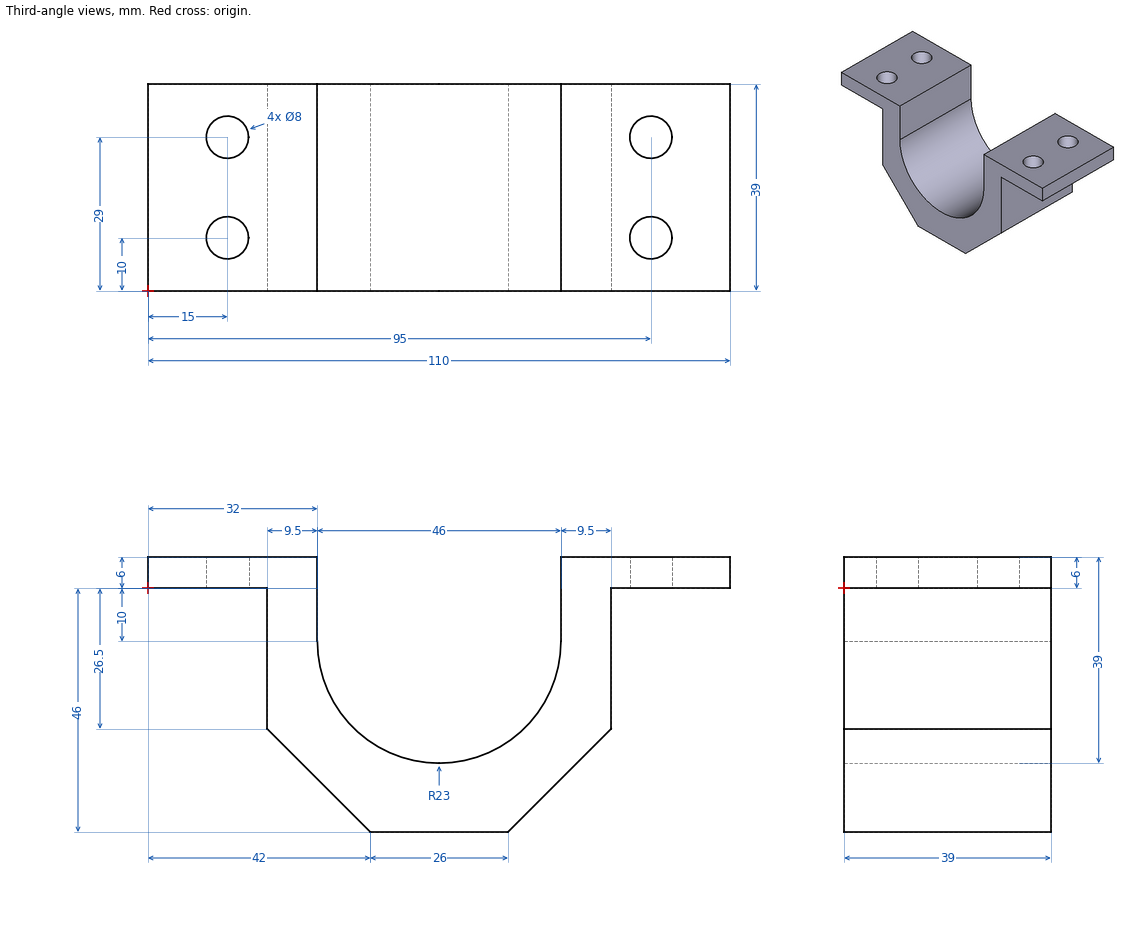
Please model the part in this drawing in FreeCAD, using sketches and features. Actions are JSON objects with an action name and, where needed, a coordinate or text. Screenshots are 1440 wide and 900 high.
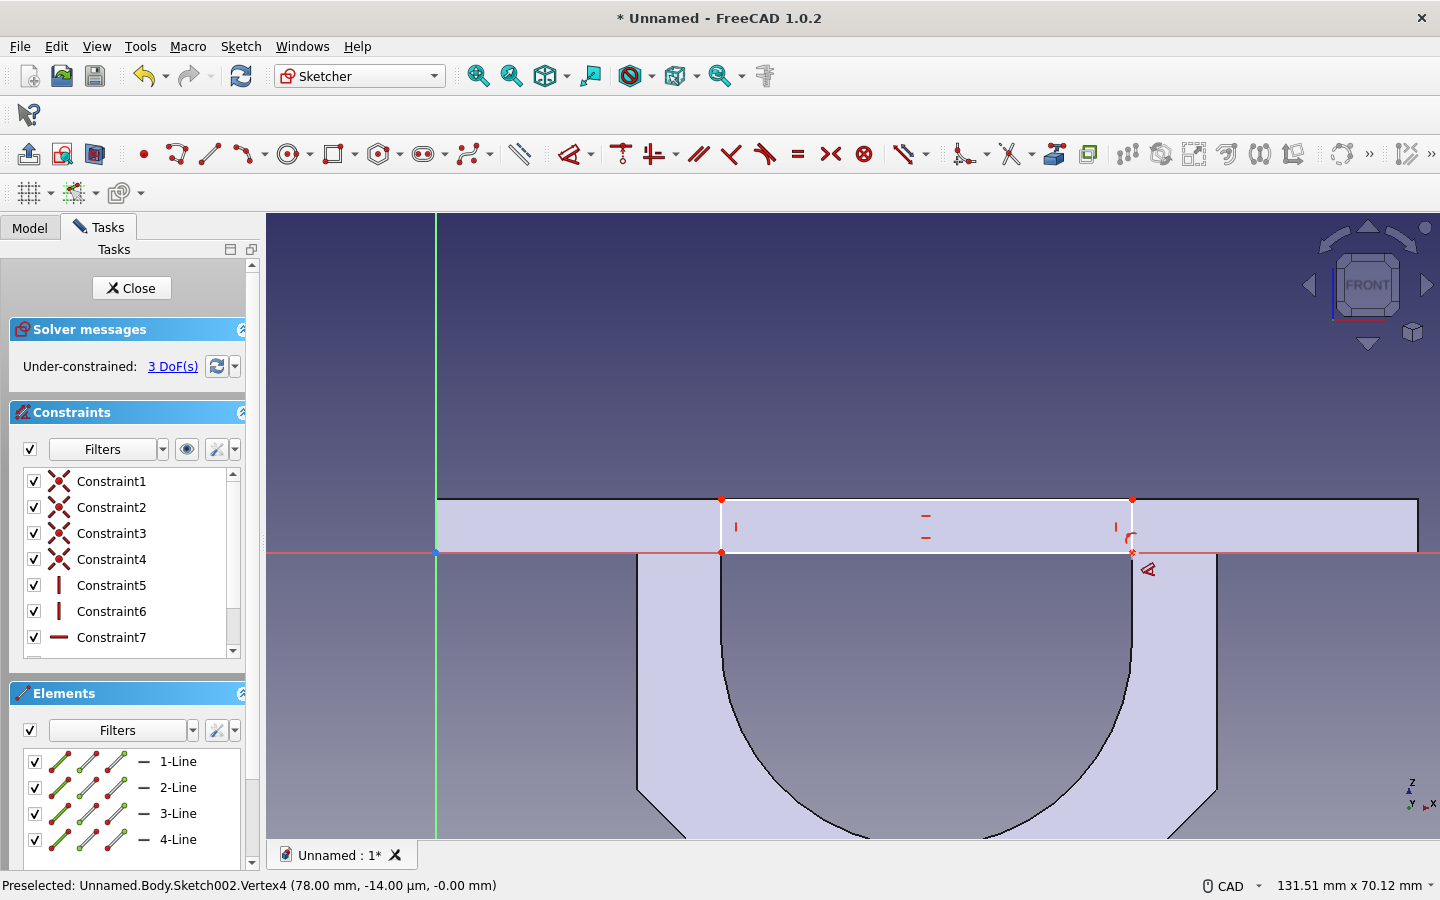
{"action": "left_click", "coordinate": [721, 516]}
{"action": "left_click", "coordinate": [687, 526]}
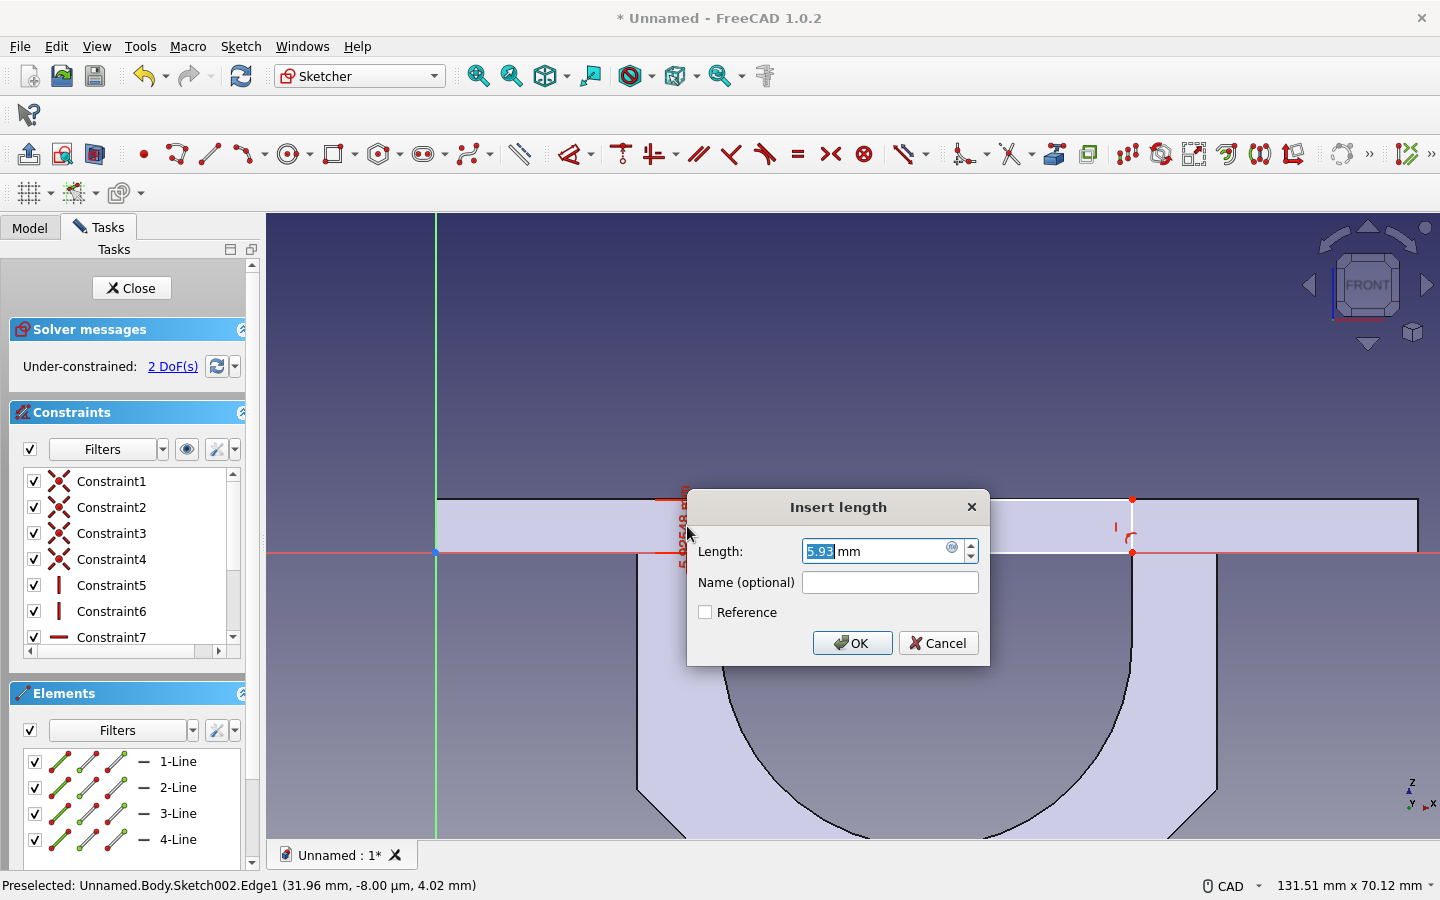
{"action": "type", "text": "6"}
{"action": "key", "text": "Return"}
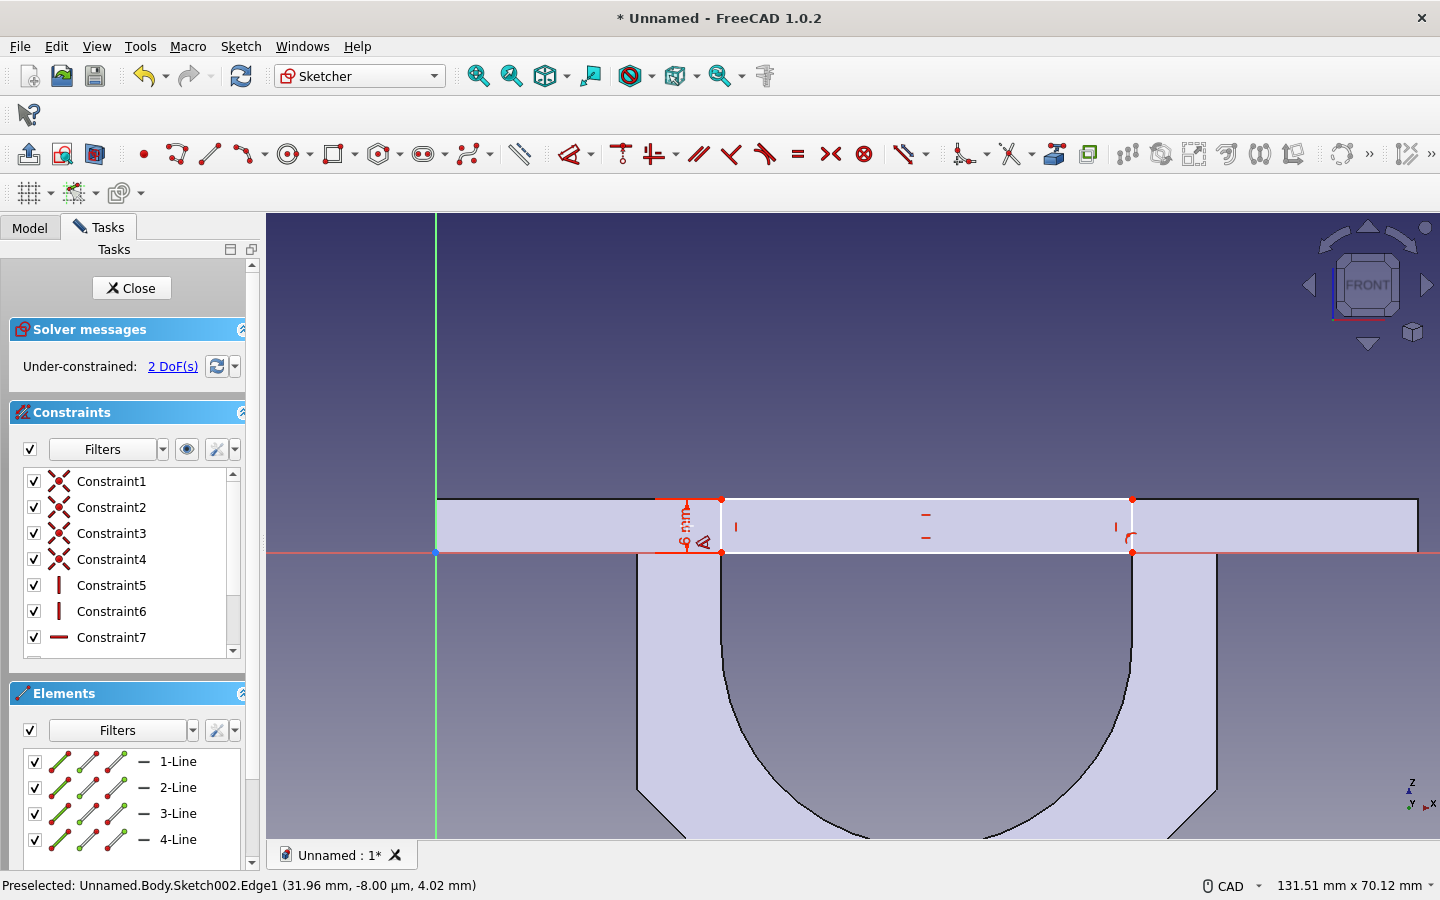
{"action": "left_click", "coordinate": [844, 553]}
{"action": "left_click", "coordinate": [926, 587]}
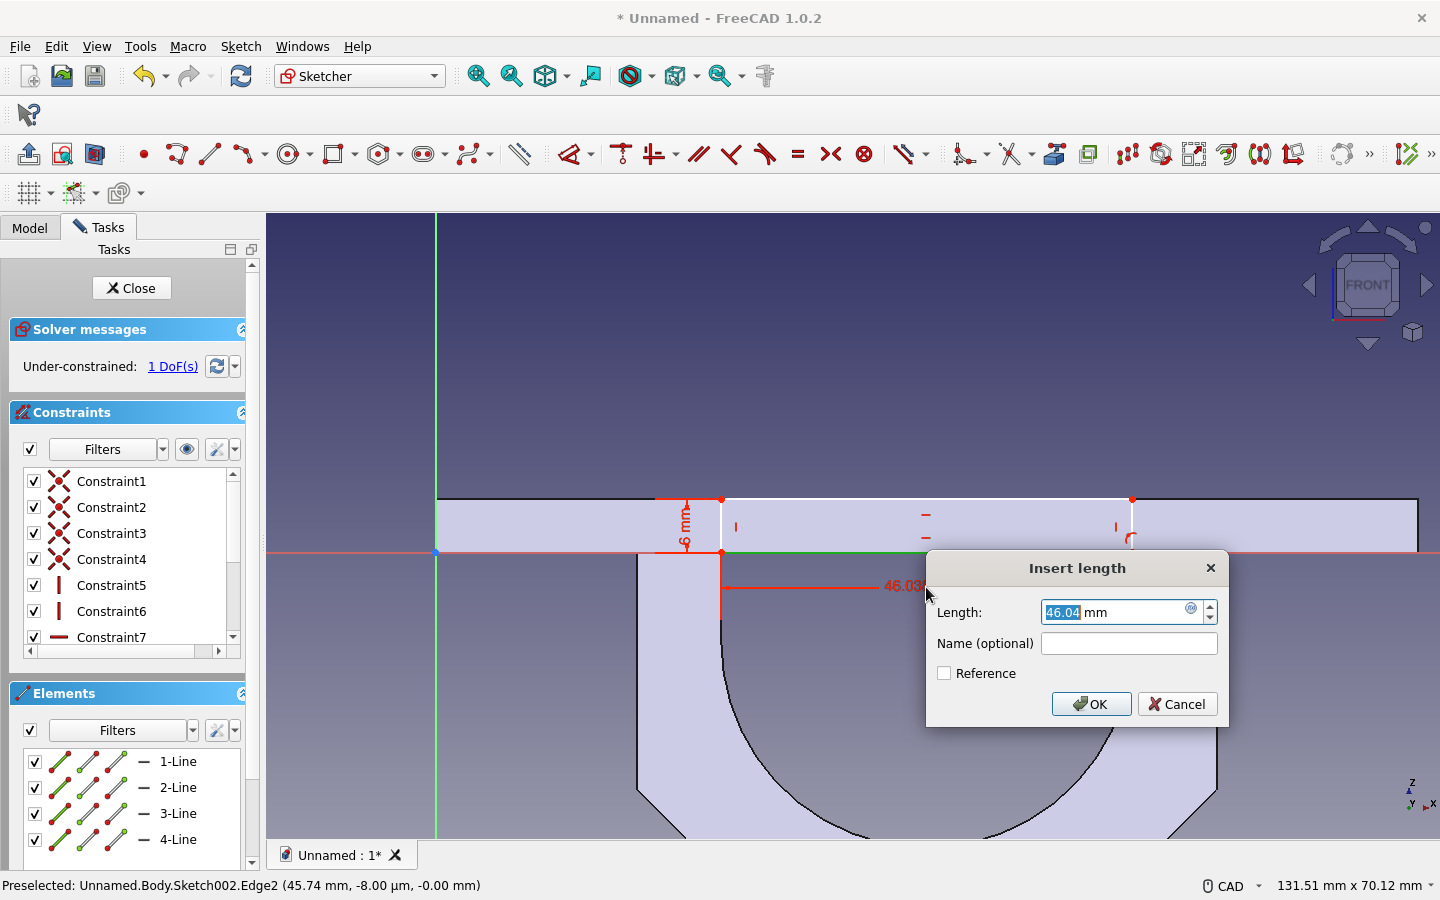
{"action": "type", "text": "46"}
{"action": "key", "text": "Return"}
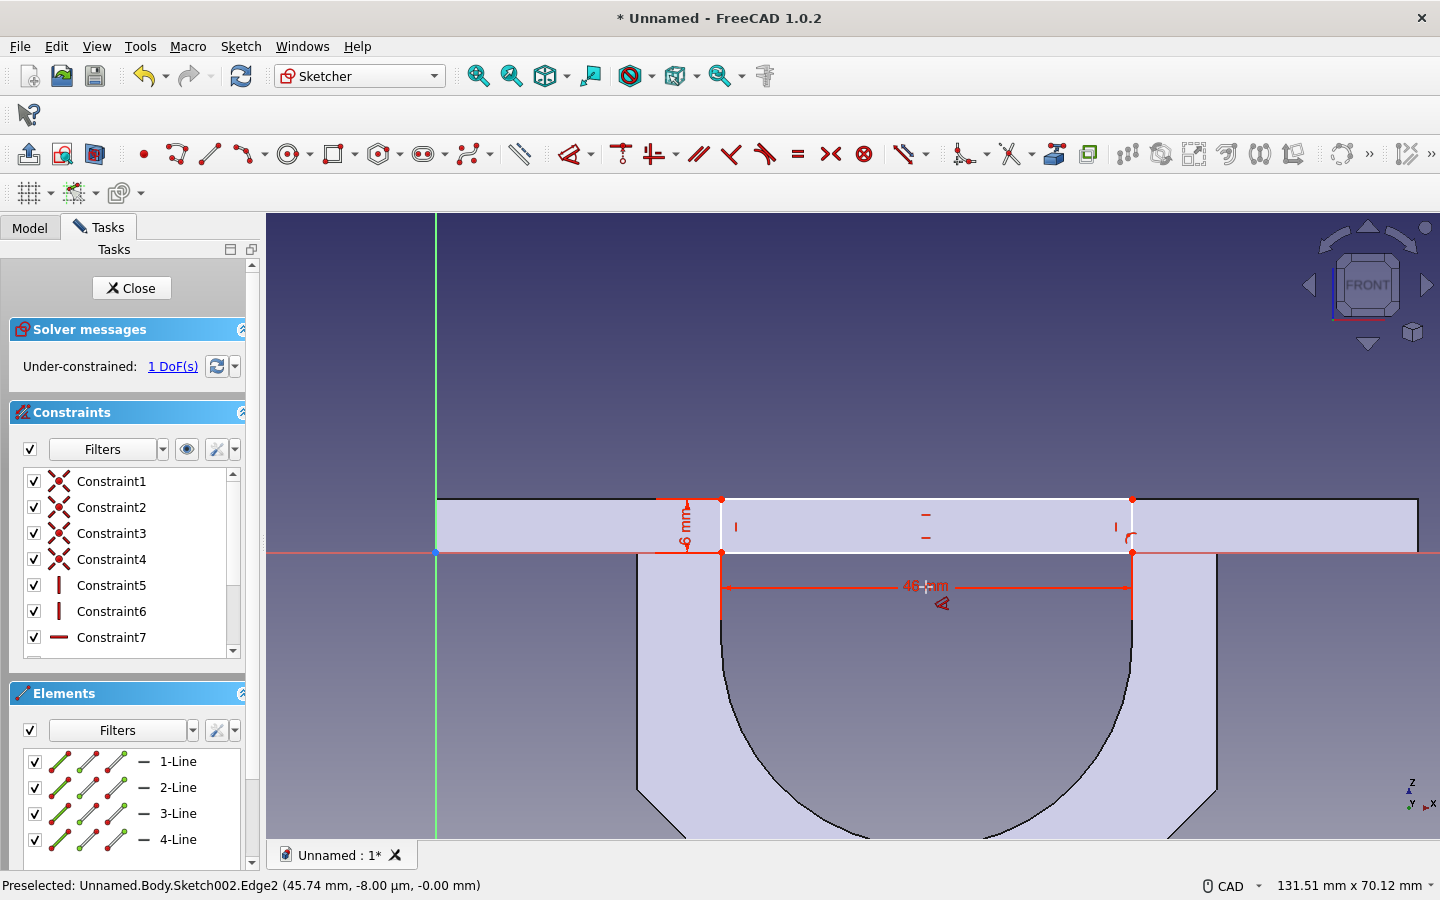
{"action": "left_click", "coordinate": [721, 499]}
{"action": "left_click", "coordinate": [578, 587]}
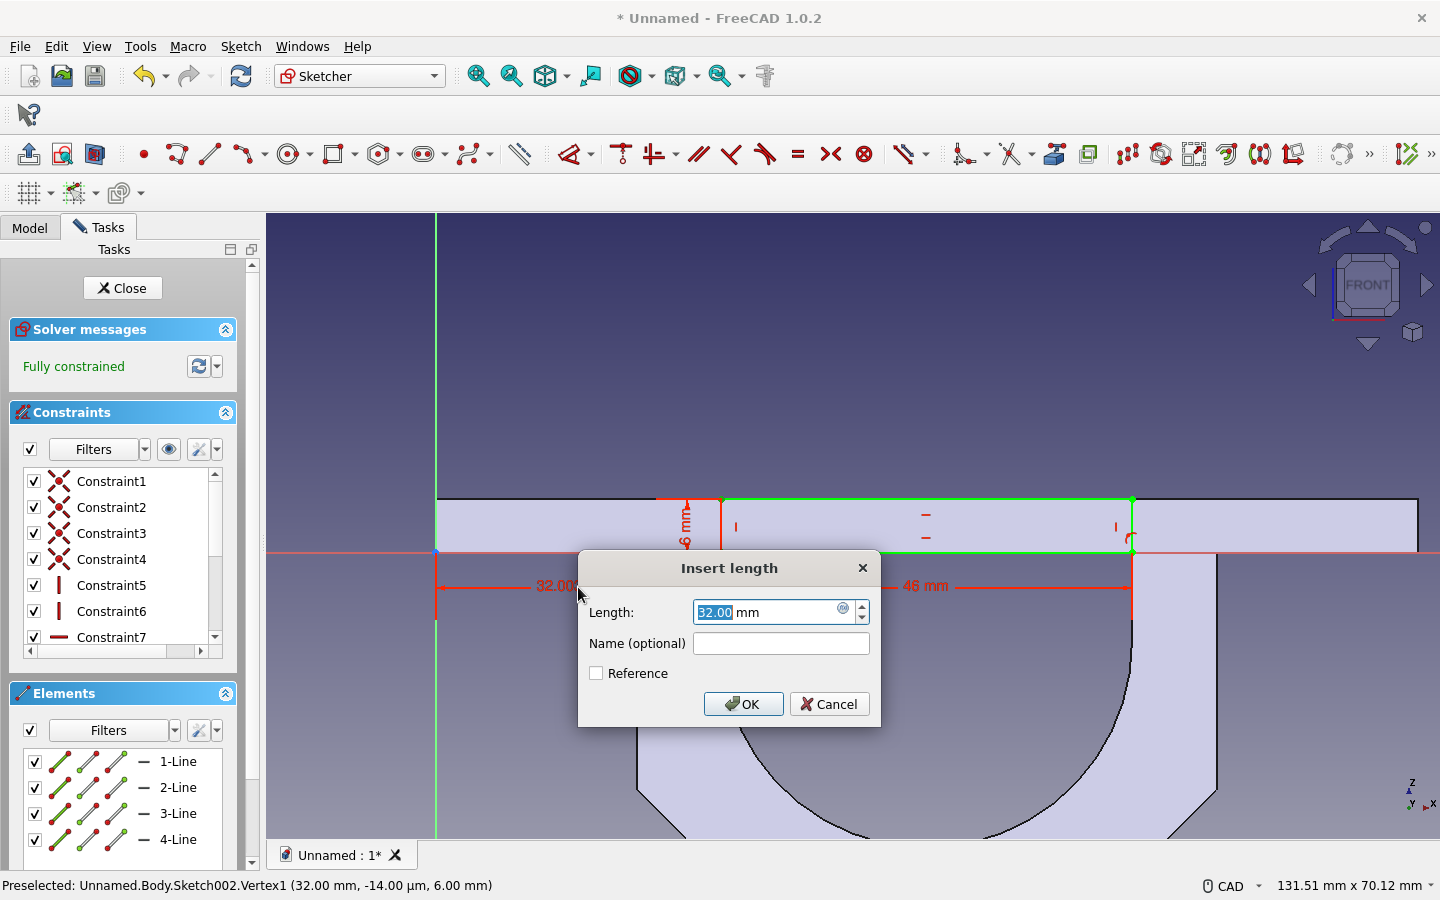
{"action": "type", "text": "32"}
{"action": "key", "text": "Return"}
{"action": "key", "text": "Escape"}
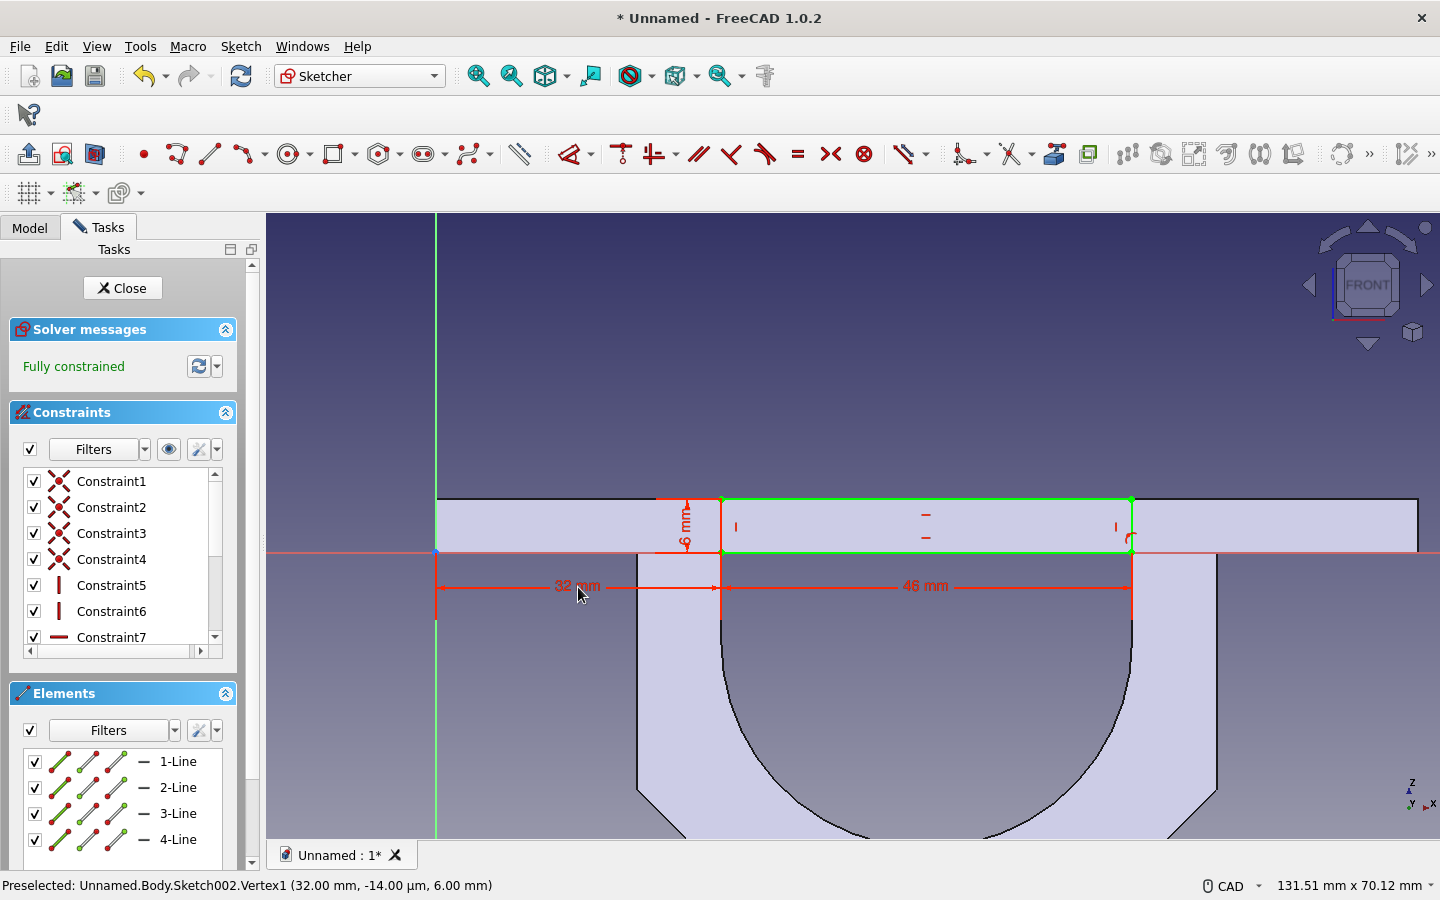
{"action": "left_click", "coordinate": [123, 288]}